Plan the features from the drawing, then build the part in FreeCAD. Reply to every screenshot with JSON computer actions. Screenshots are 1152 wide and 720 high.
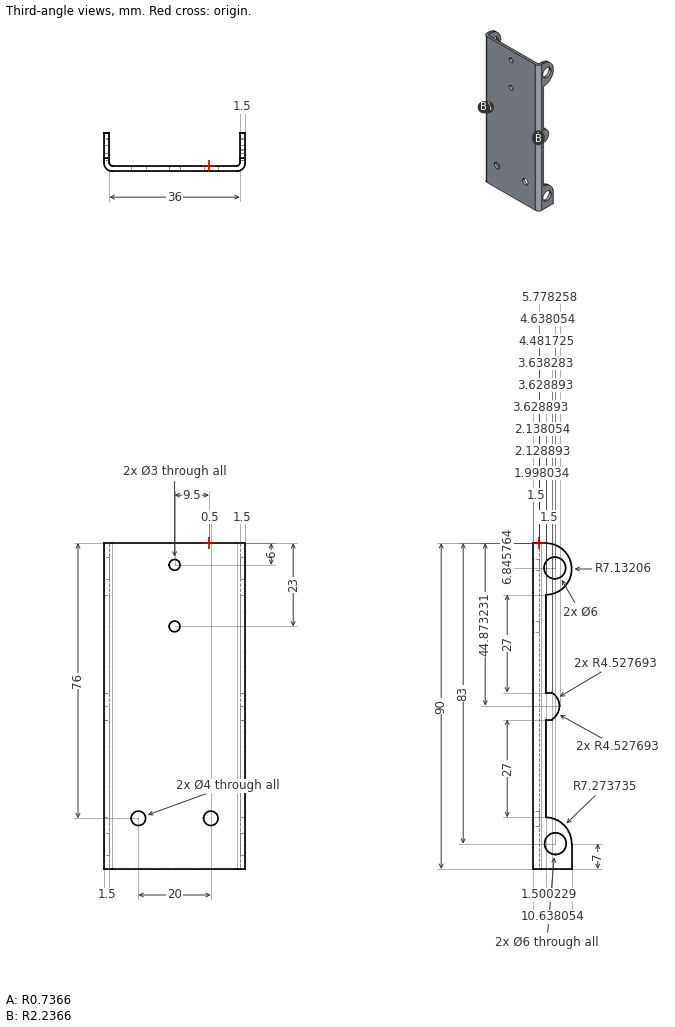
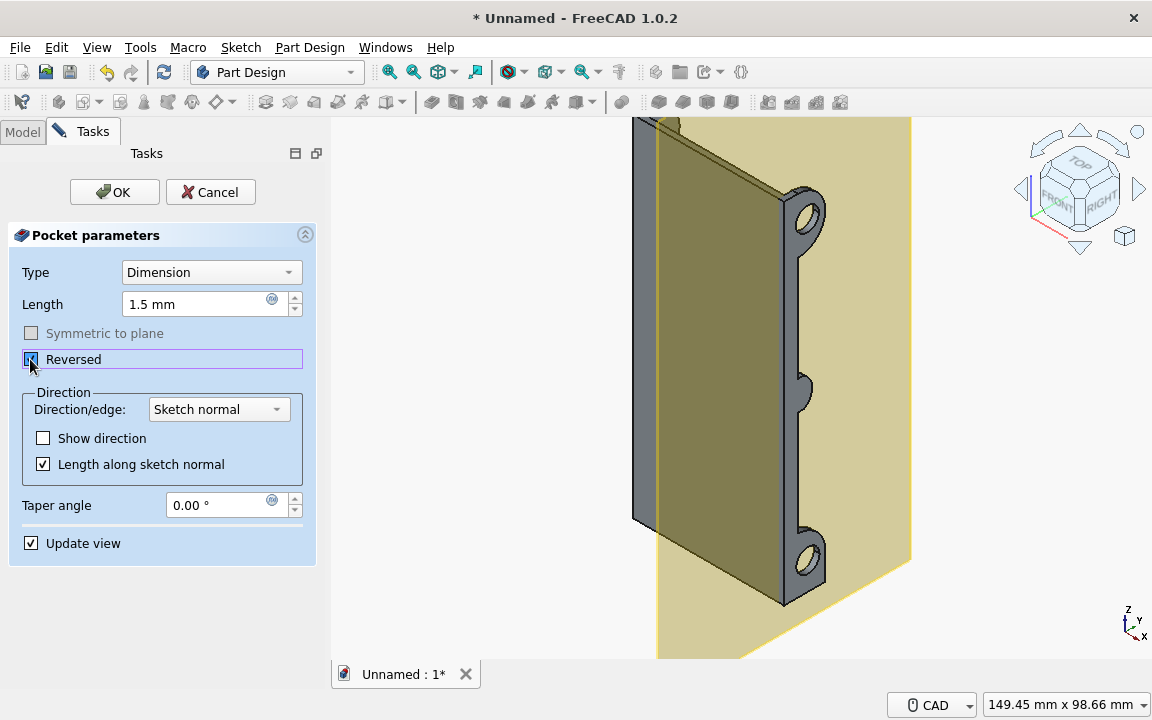
{"action": "left_click", "coordinate": [115, 192]}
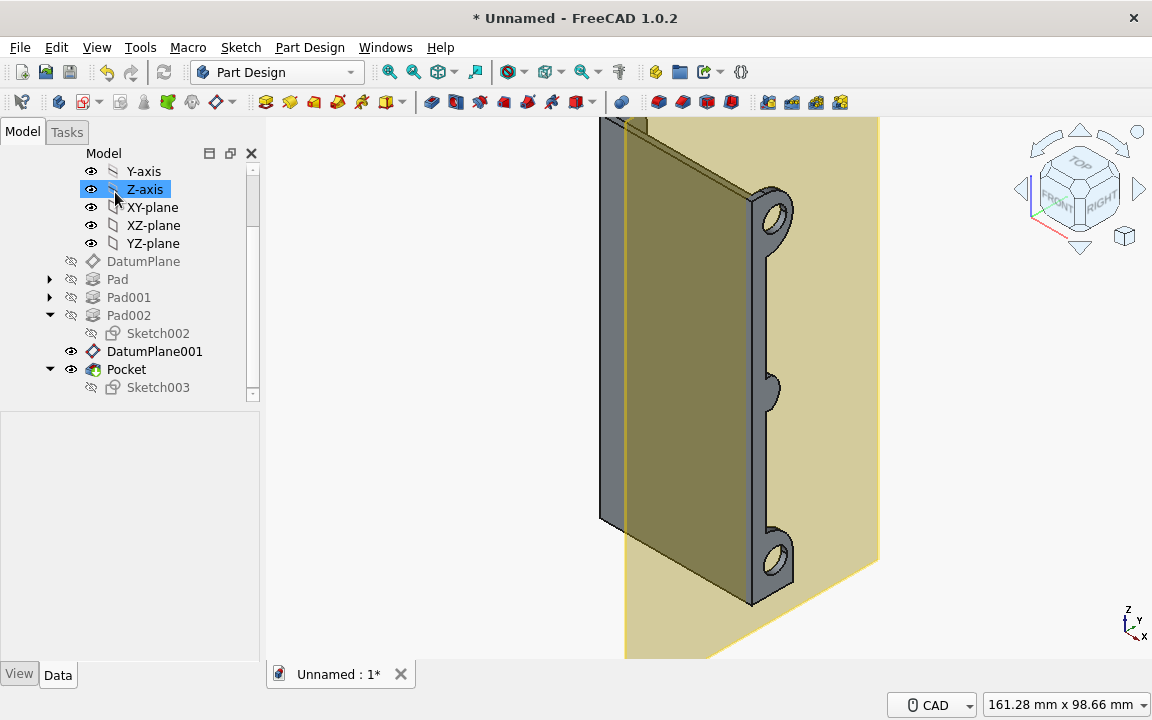
{"action": "left_click", "coordinate": [116, 351]}
{"action": "key", "text": "space"}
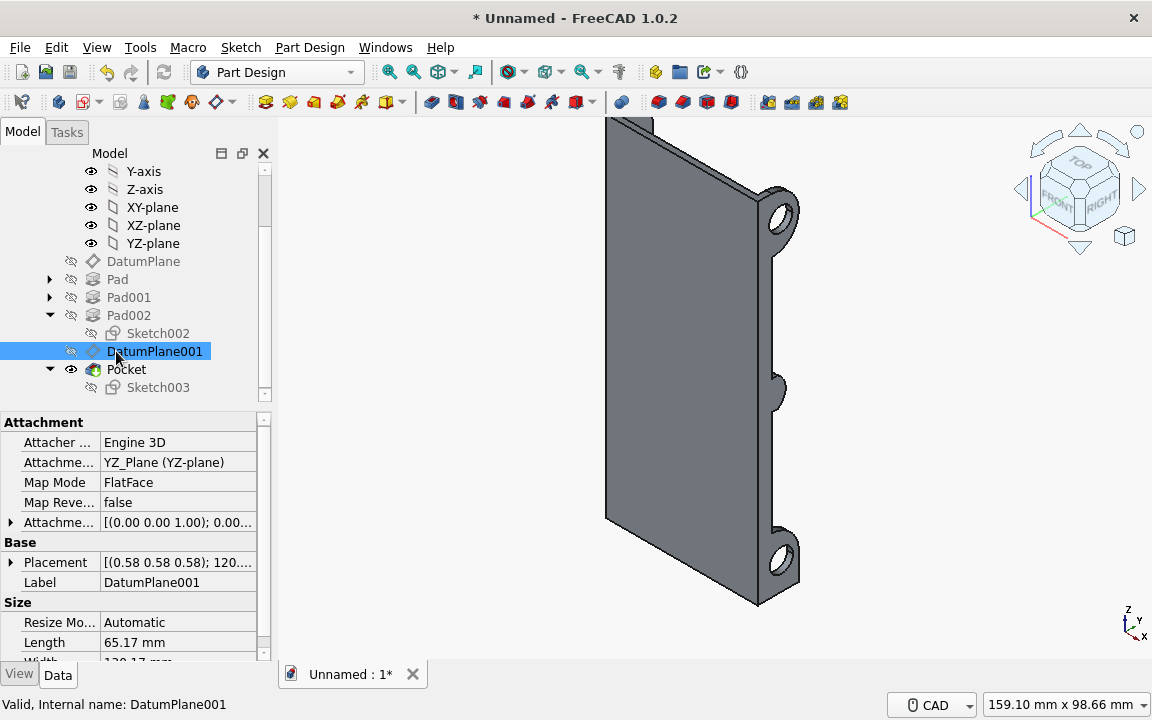
{"action": "left_click", "coordinate": [390, 72]}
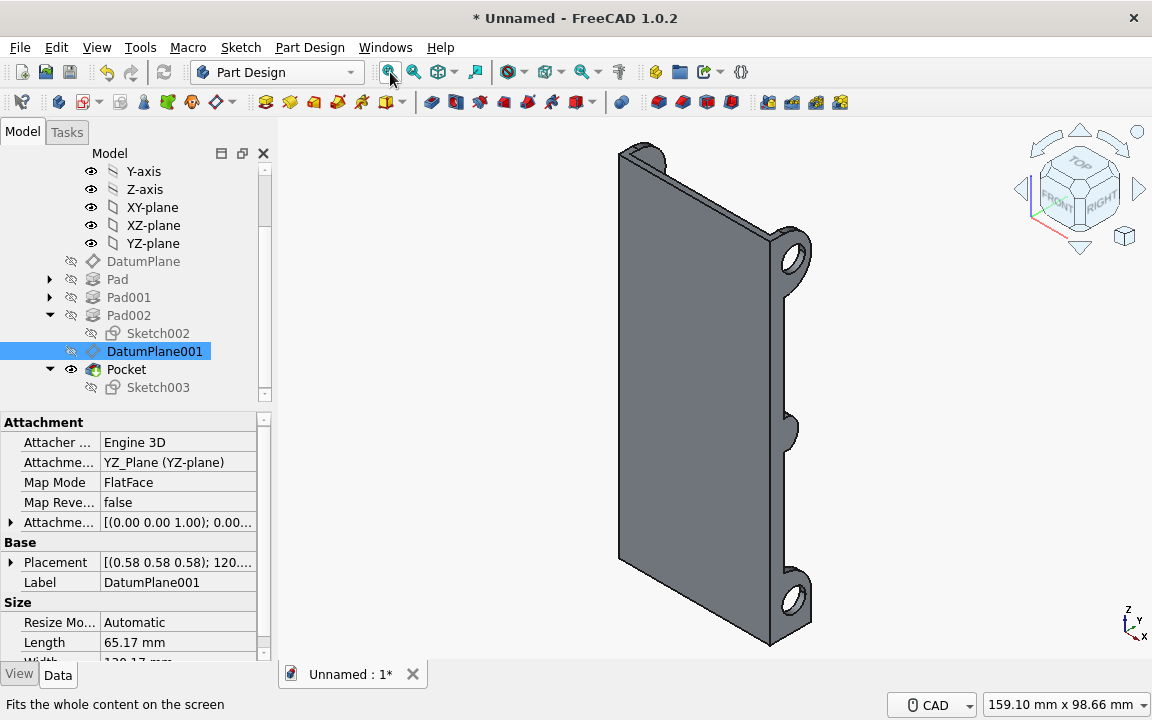
{"action": "key", "text": "3"}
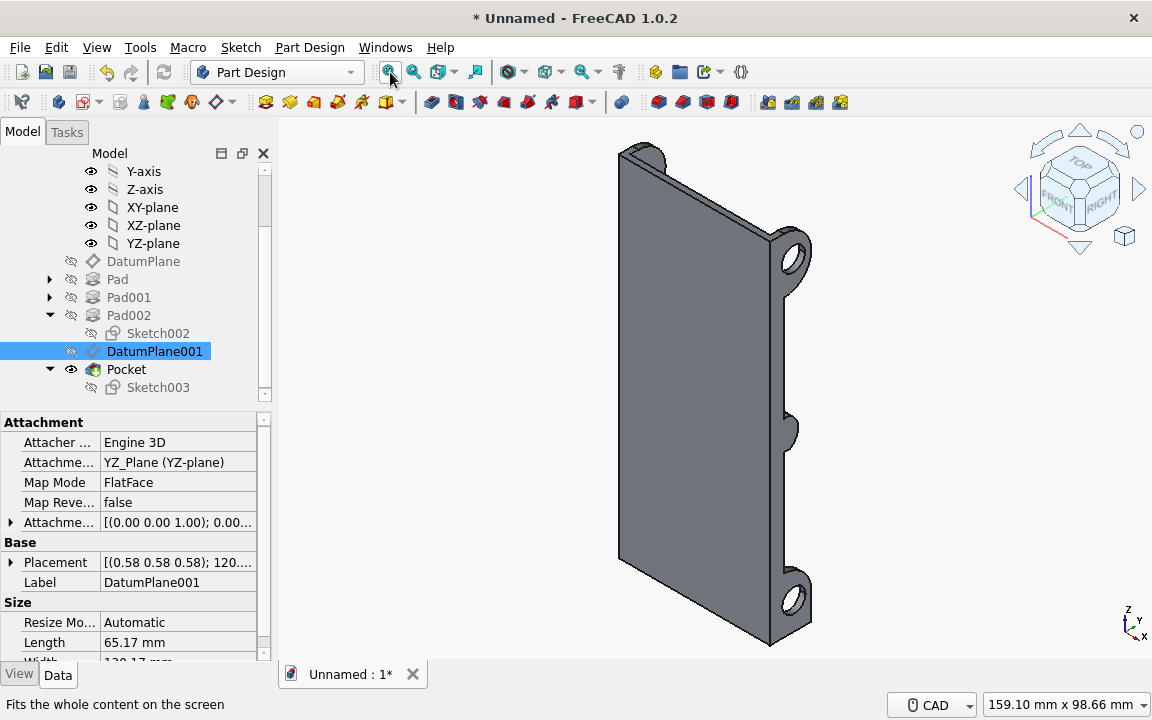
{"action": "left_click", "coordinate": [719, 599]}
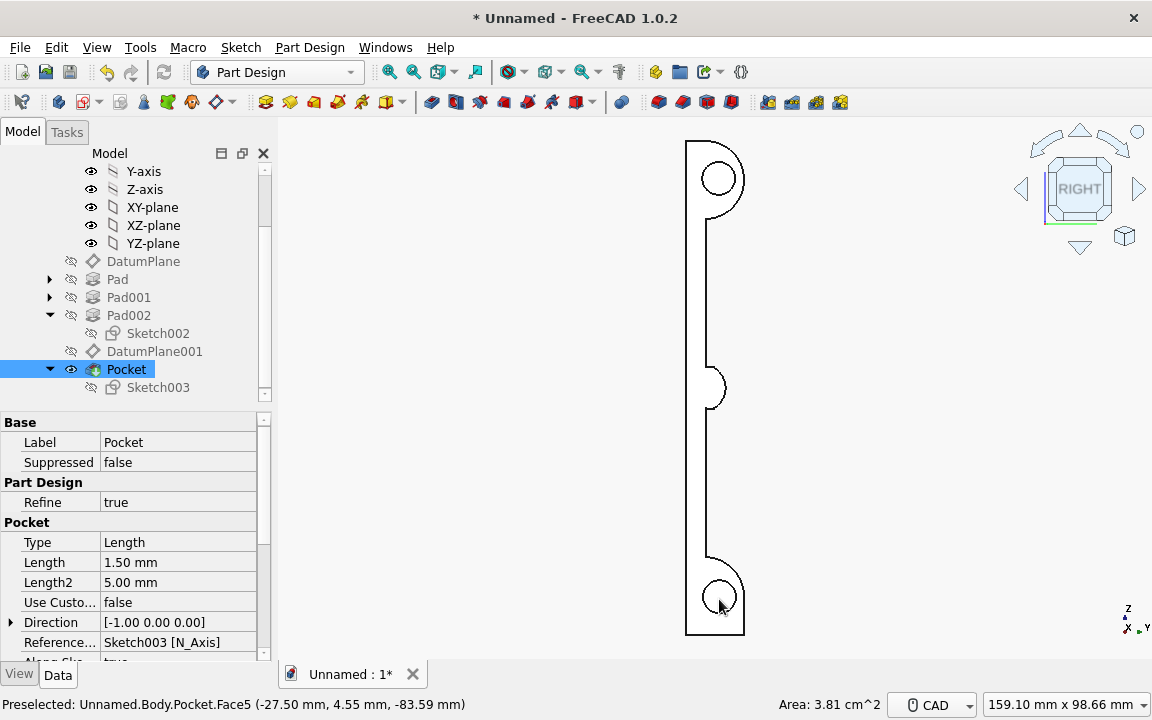
{"action": "left_click", "coordinate": [84, 102]}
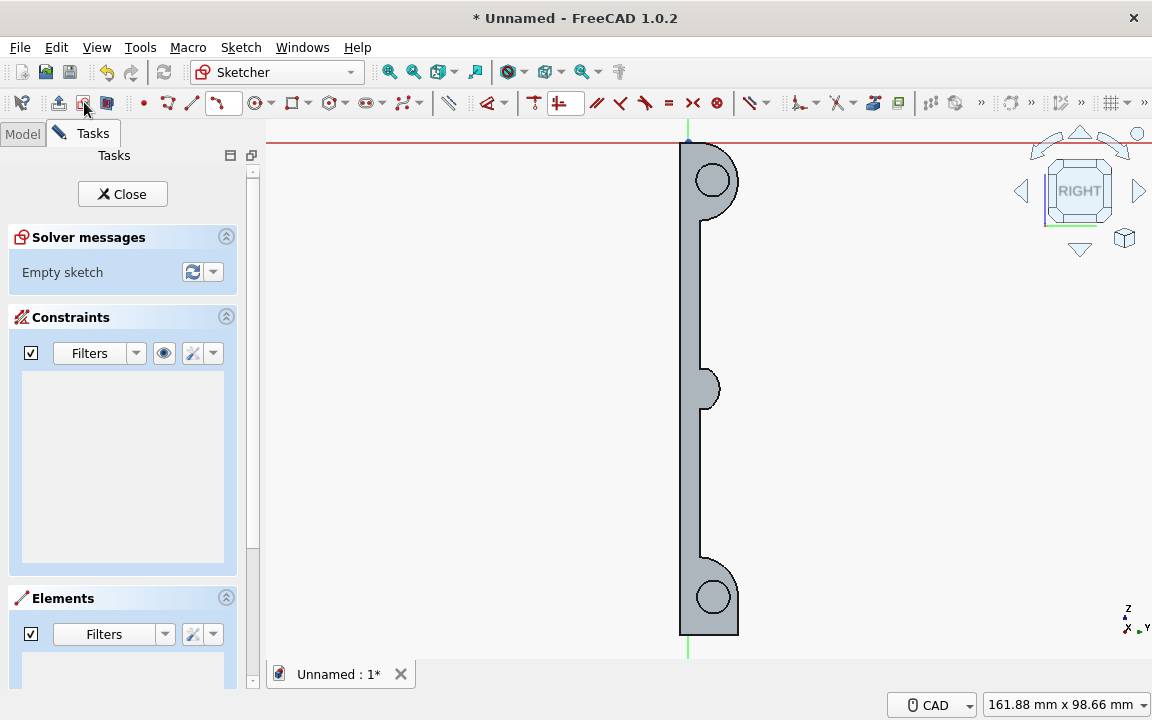
{"action": "scroll", "coordinate": [501, 411], "scroll_direction": "down", "scroll_amount": 2}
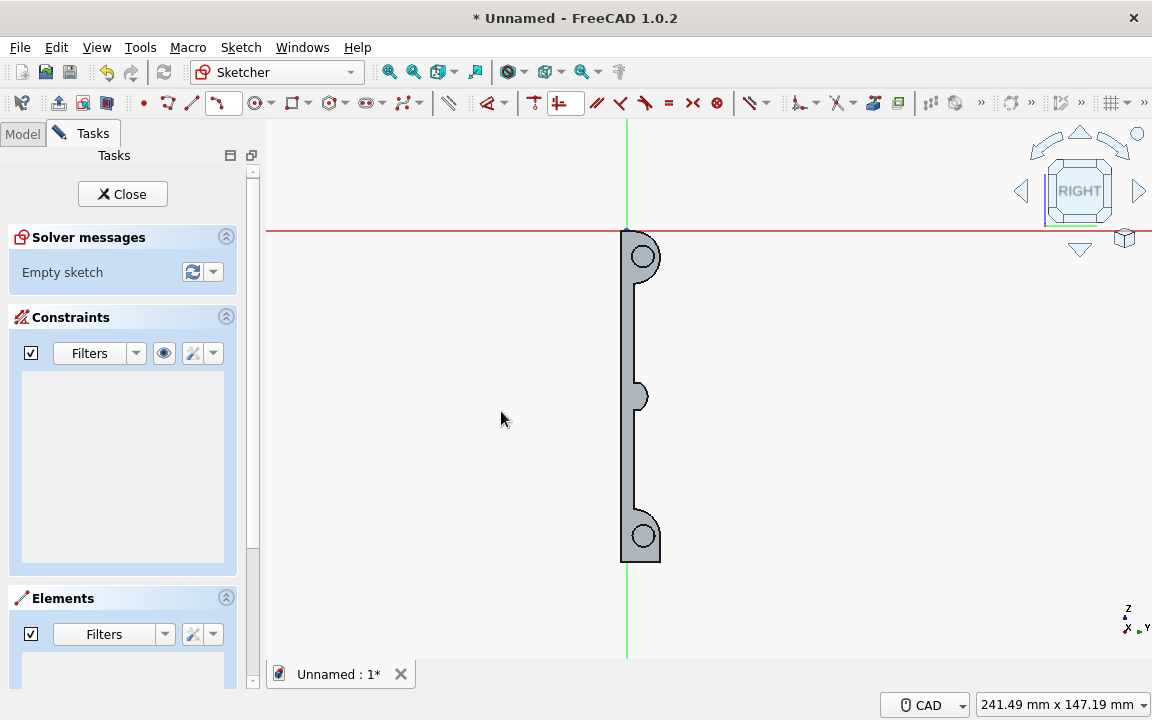
{"action": "key", "text": "g c"}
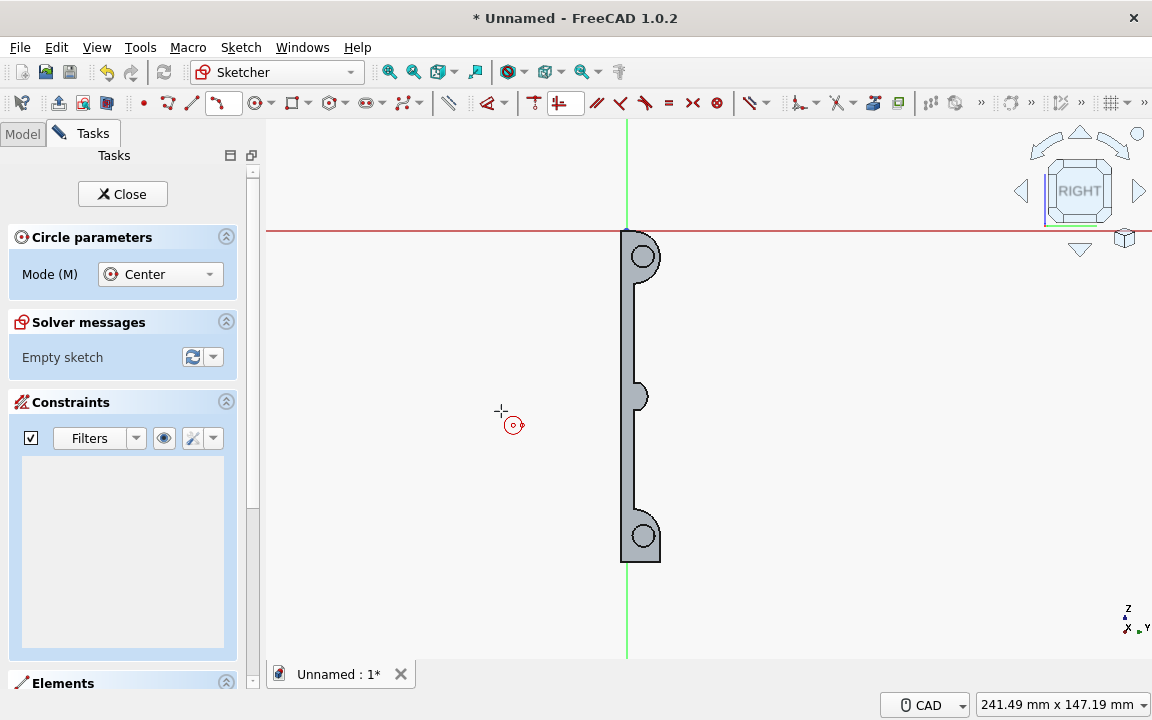
{"action": "scroll", "coordinate": [644, 536], "scroll_direction": "up", "scroll_amount": 4}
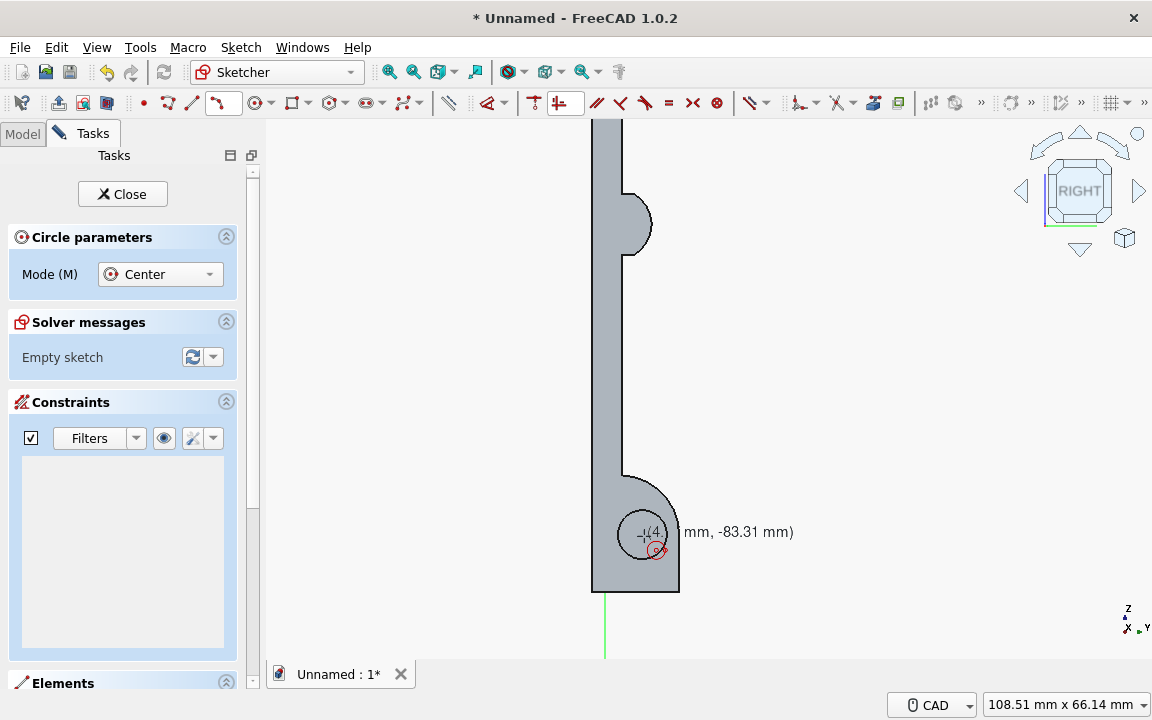
{"action": "left_click", "coordinate": [642, 535]}
{"action": "left_click", "coordinate": [660, 517]}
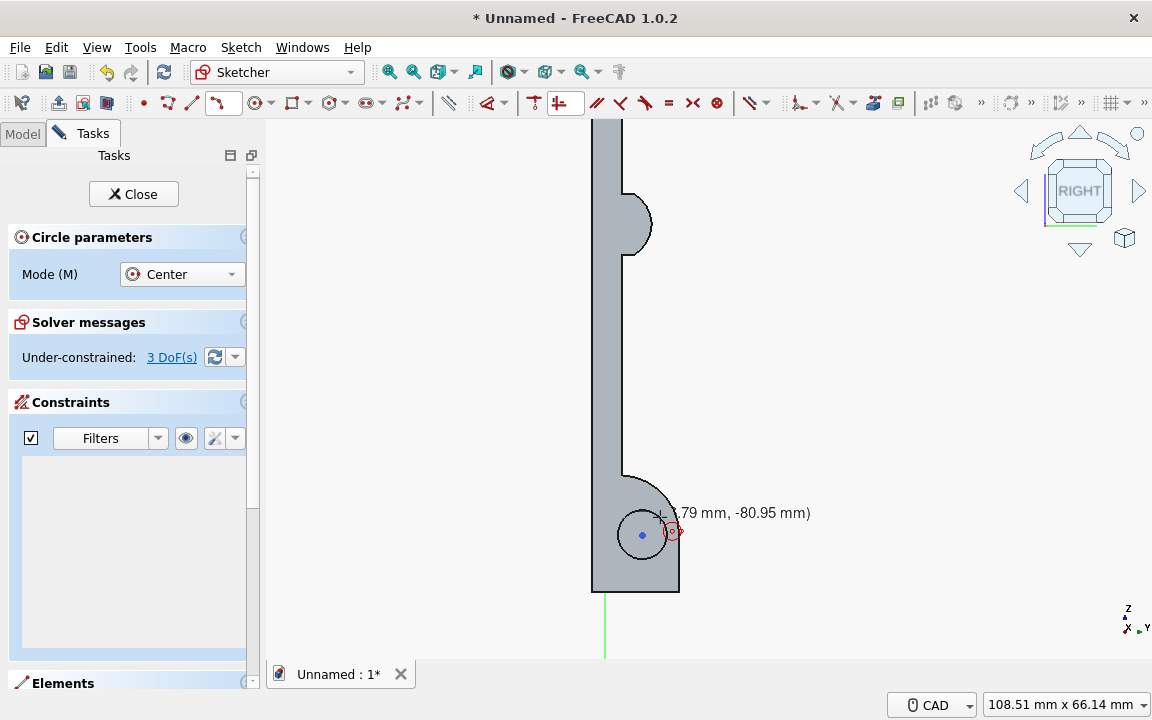
{"action": "scroll", "coordinate": [644, 537], "scroll_direction": "down", "scroll_amount": 4}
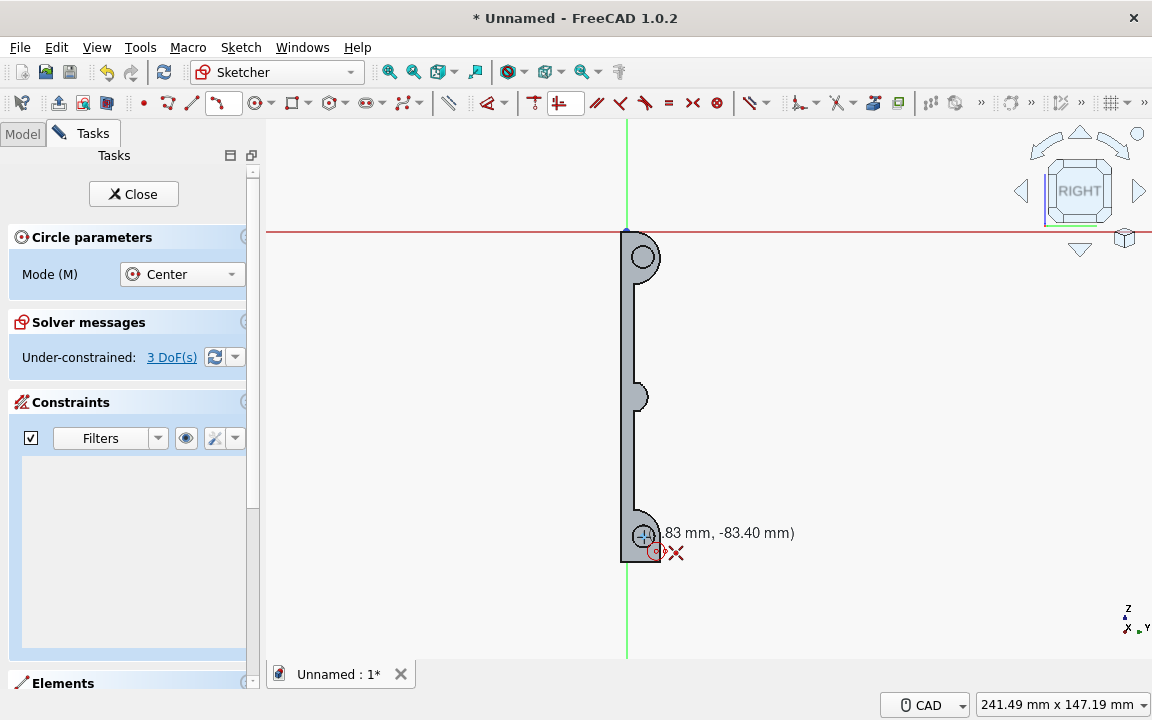
{"action": "scroll", "coordinate": [643, 257], "scroll_direction": "up", "scroll_amount": 4}